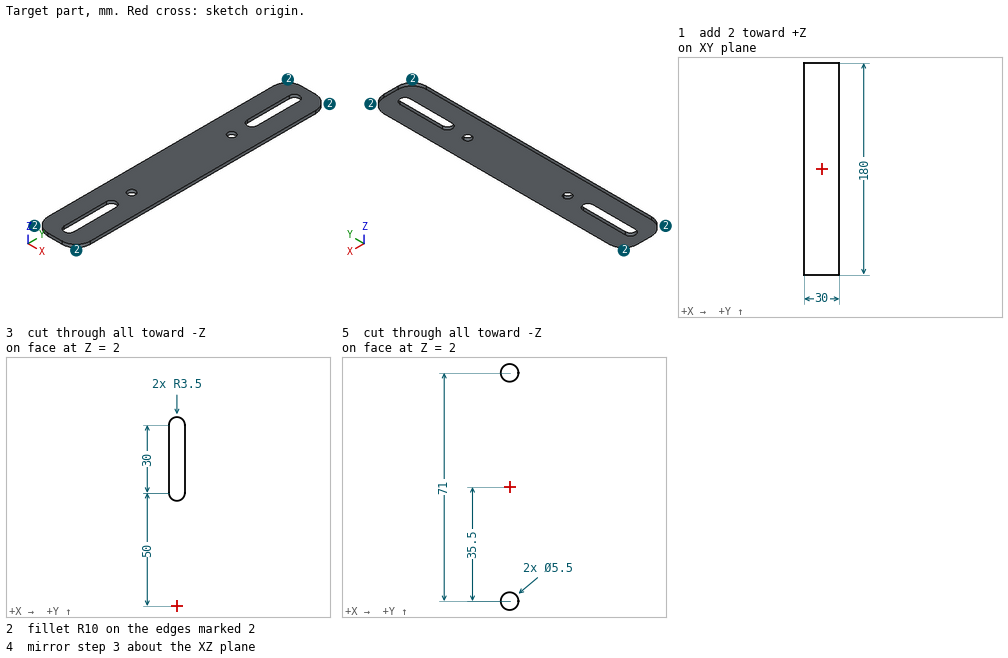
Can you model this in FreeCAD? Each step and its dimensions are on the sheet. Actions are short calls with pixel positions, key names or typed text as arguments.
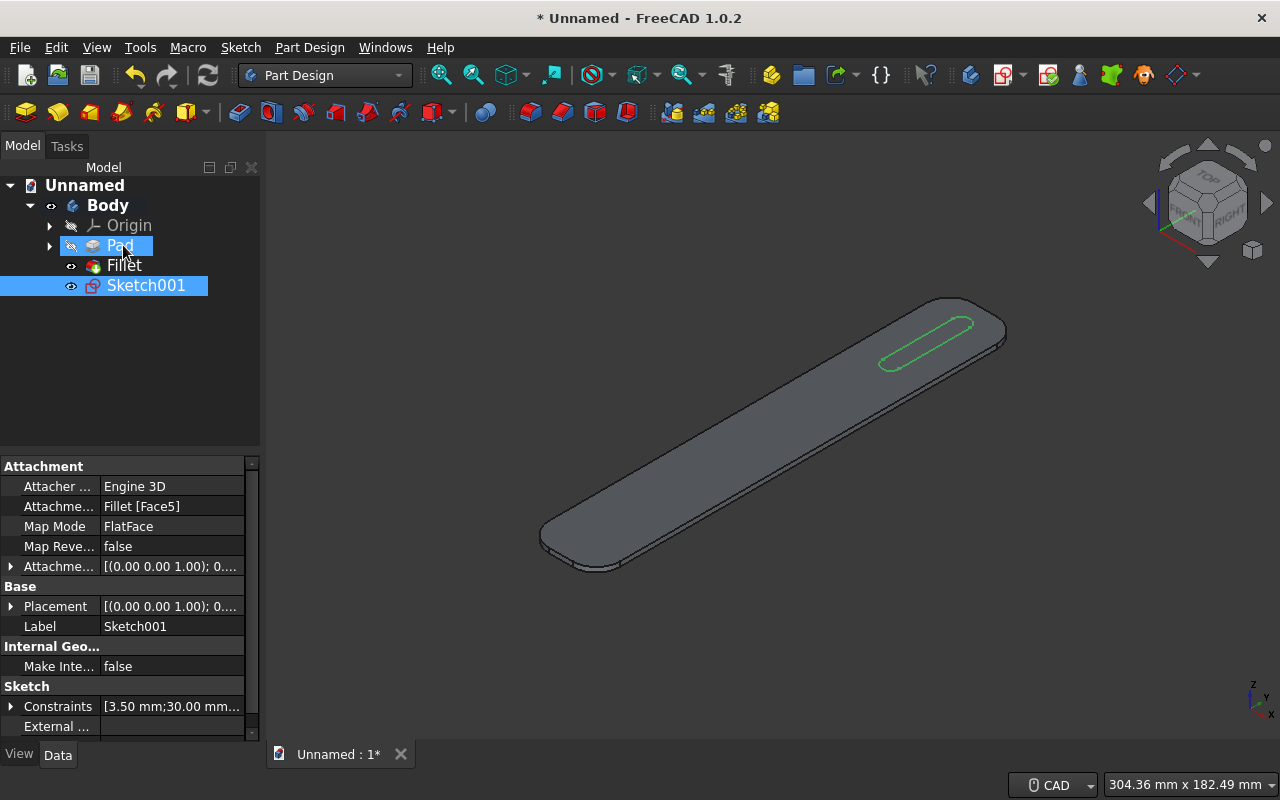
click(240, 112)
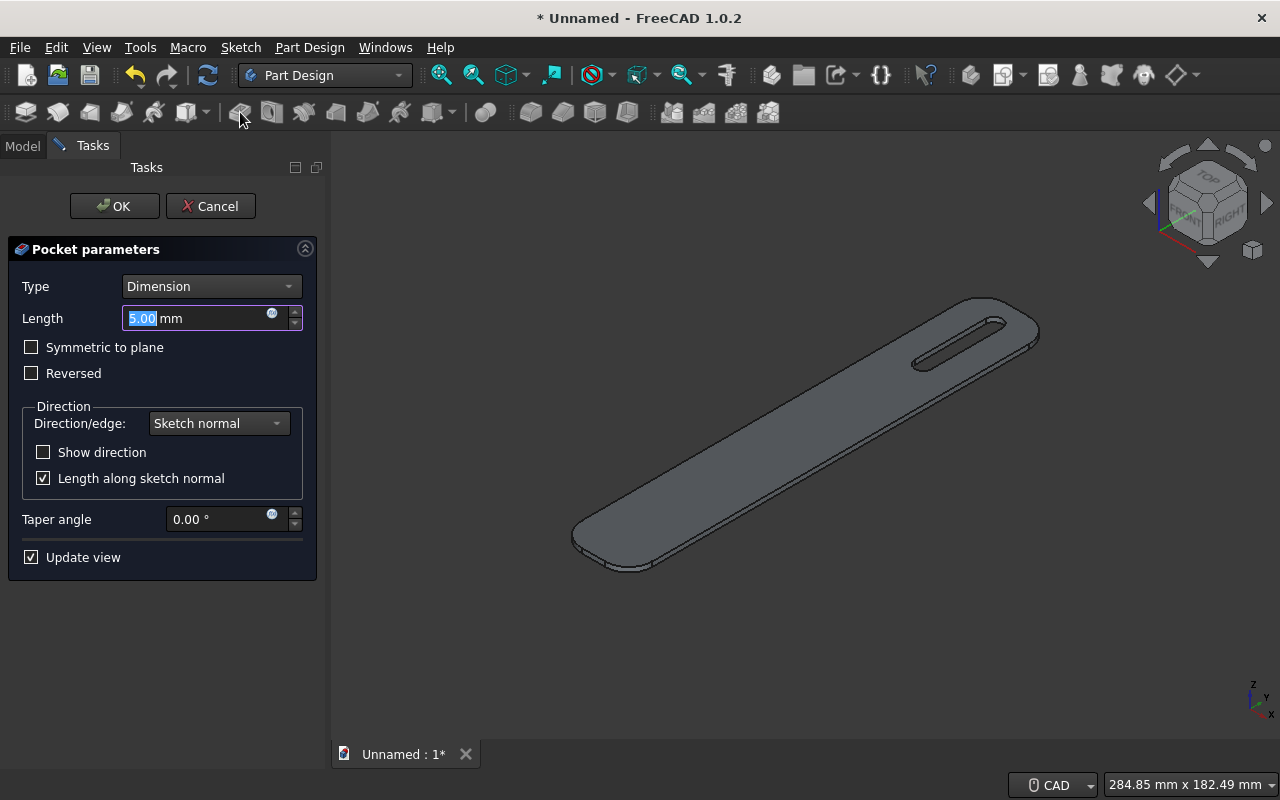
click(212, 286)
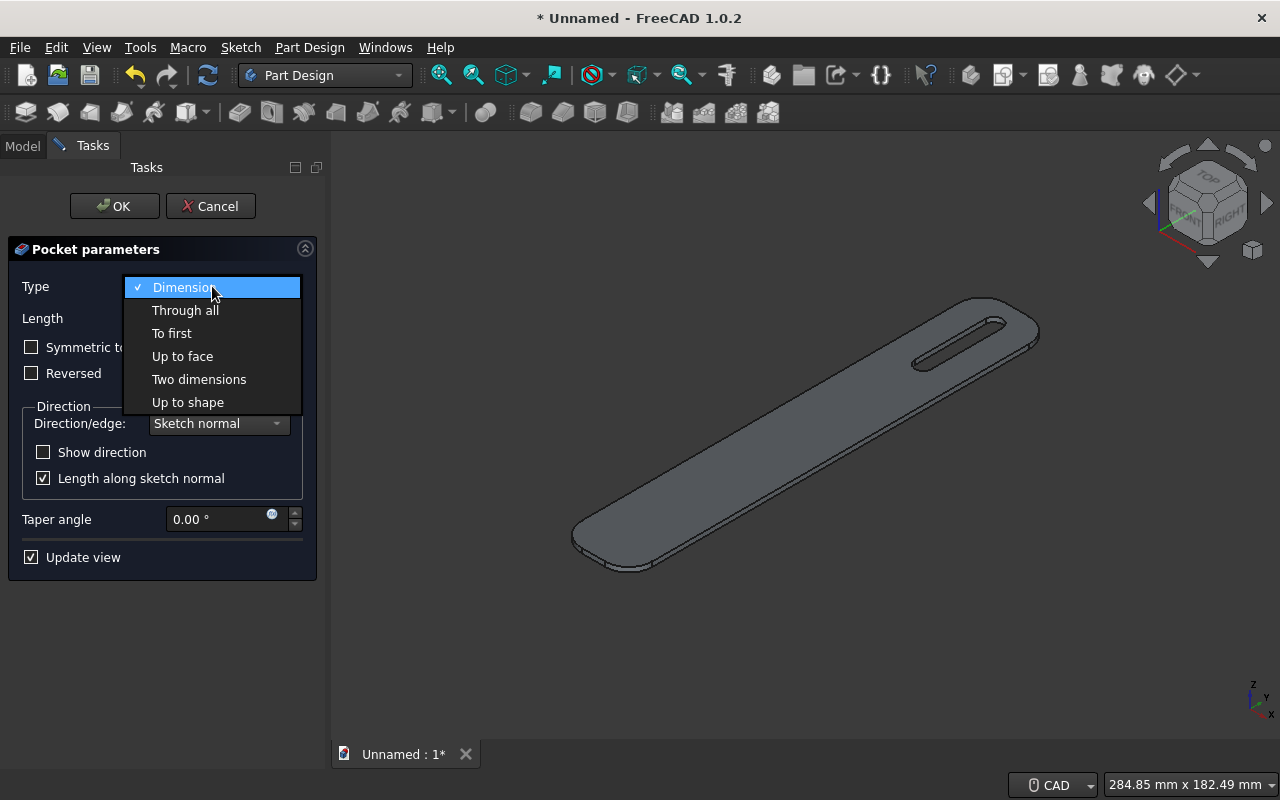
click(212, 310)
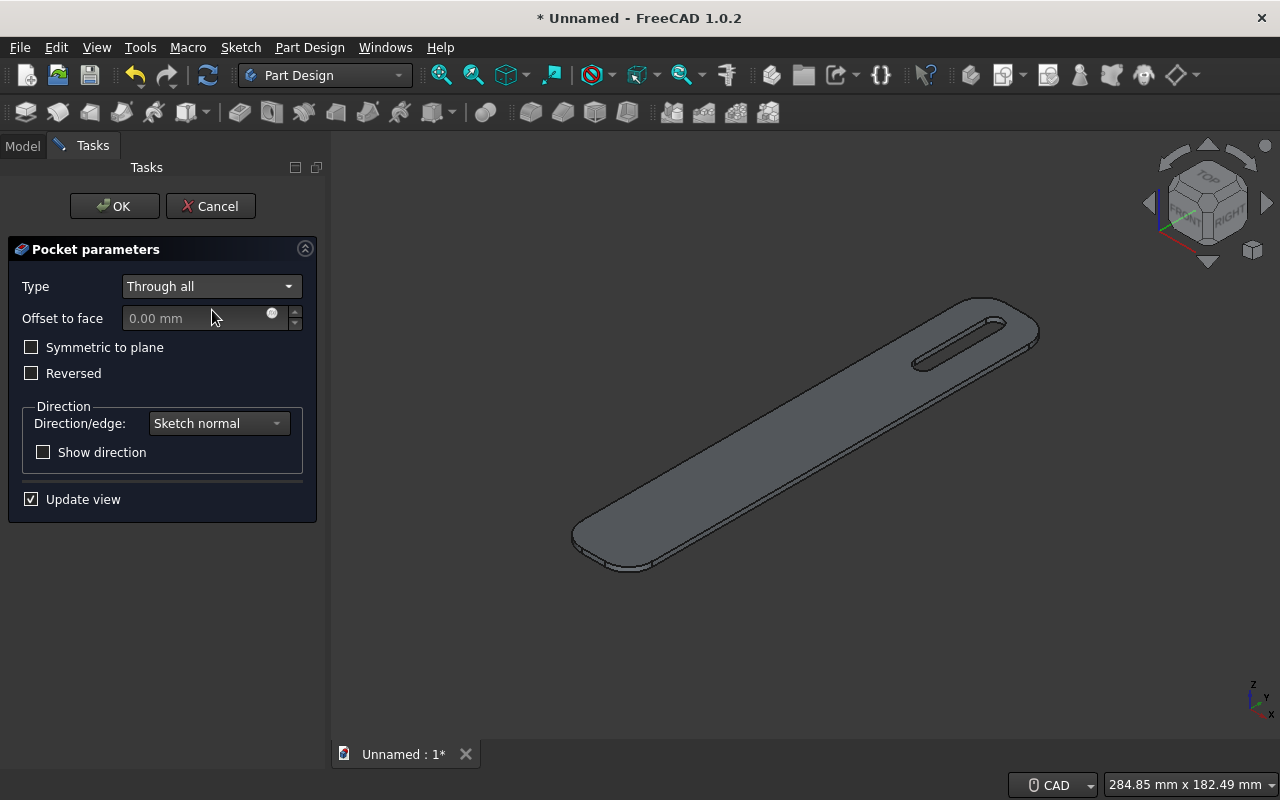
click(115, 206)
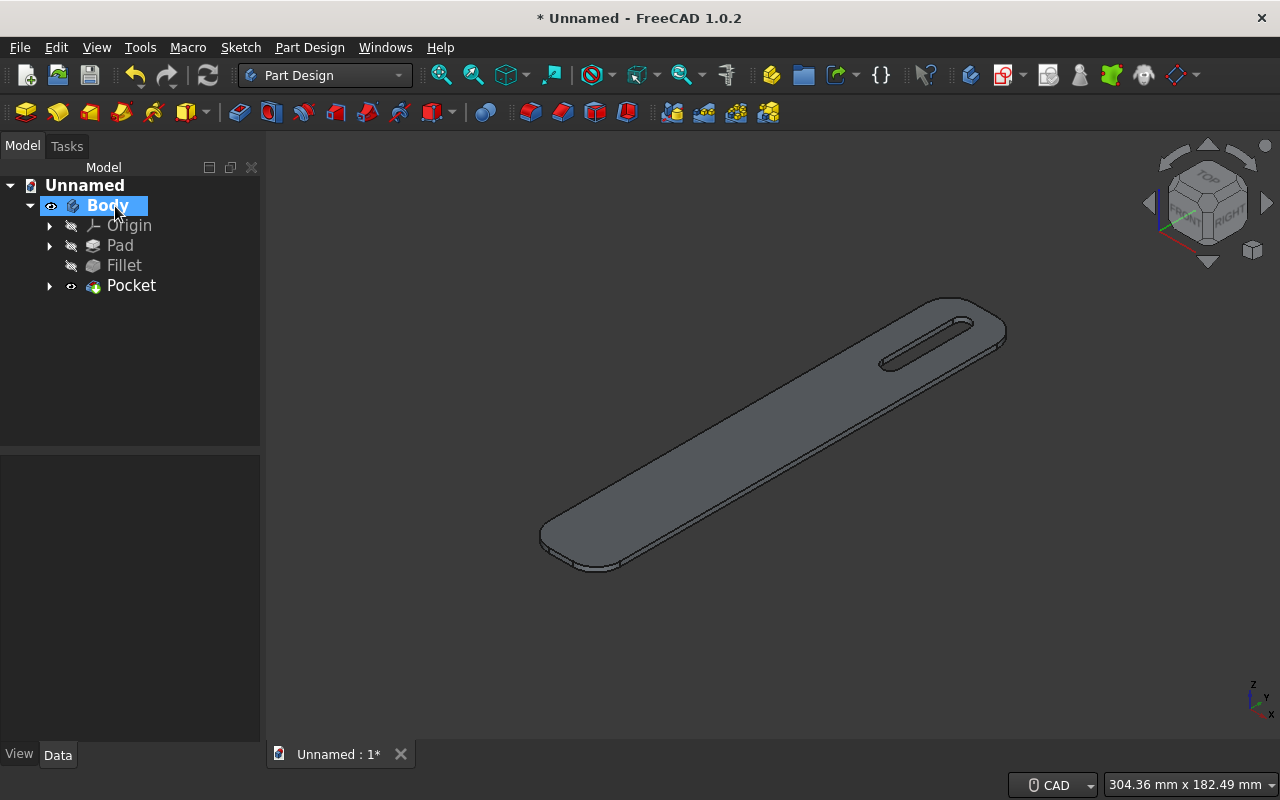
click(116, 286)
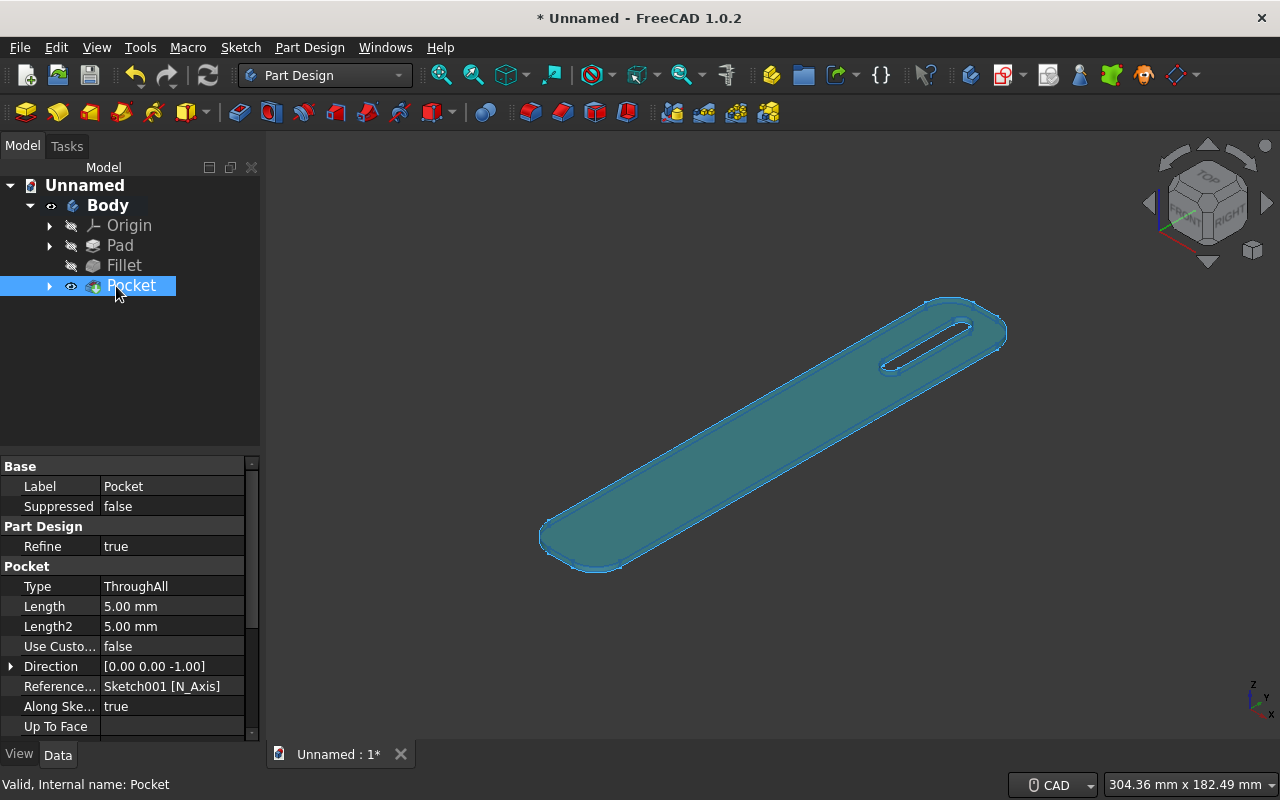
click(672, 112)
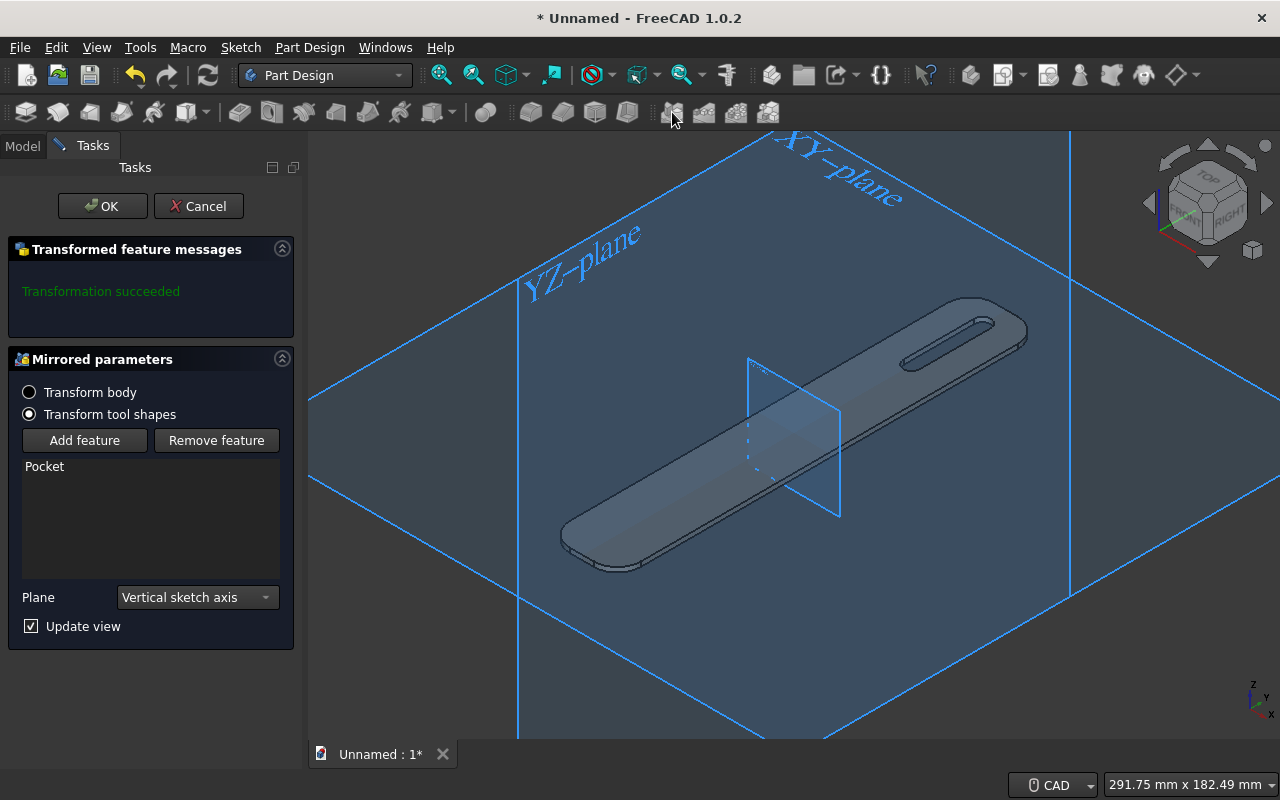
click(198, 598)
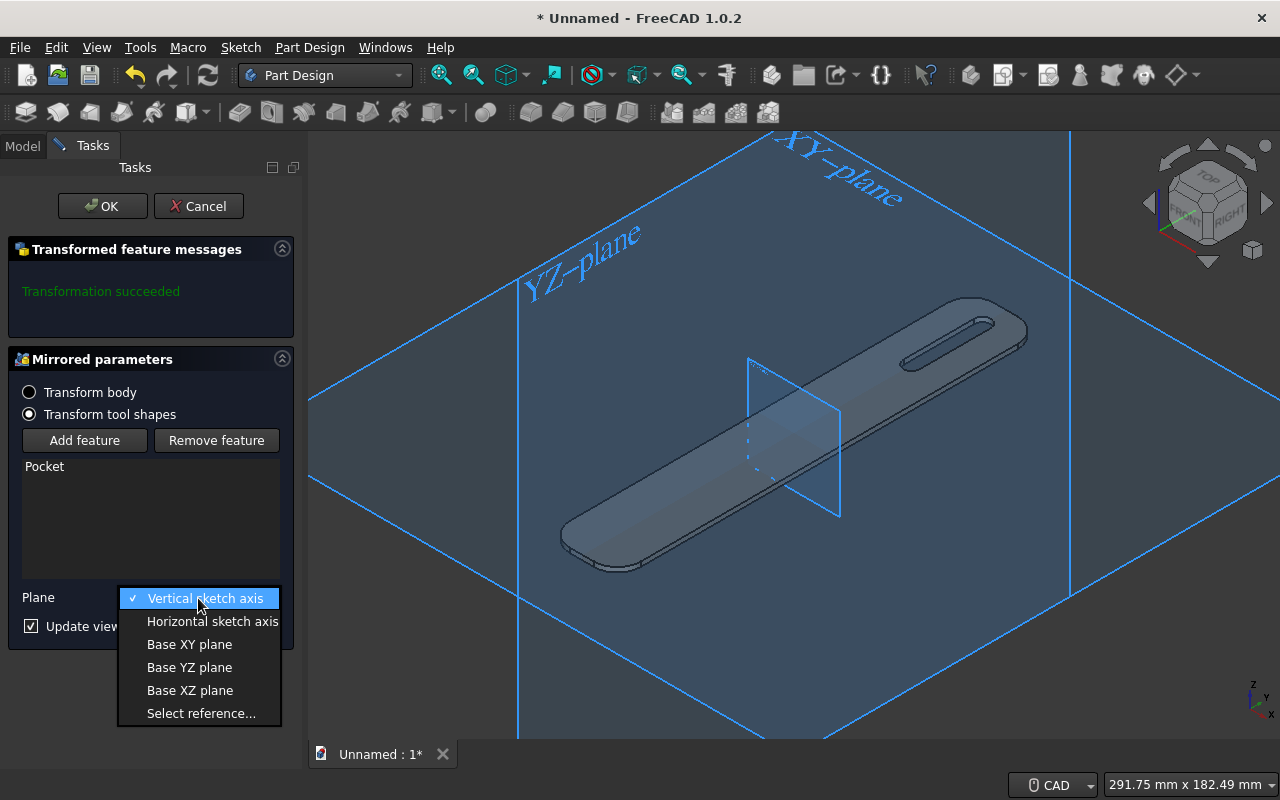
click(198, 690)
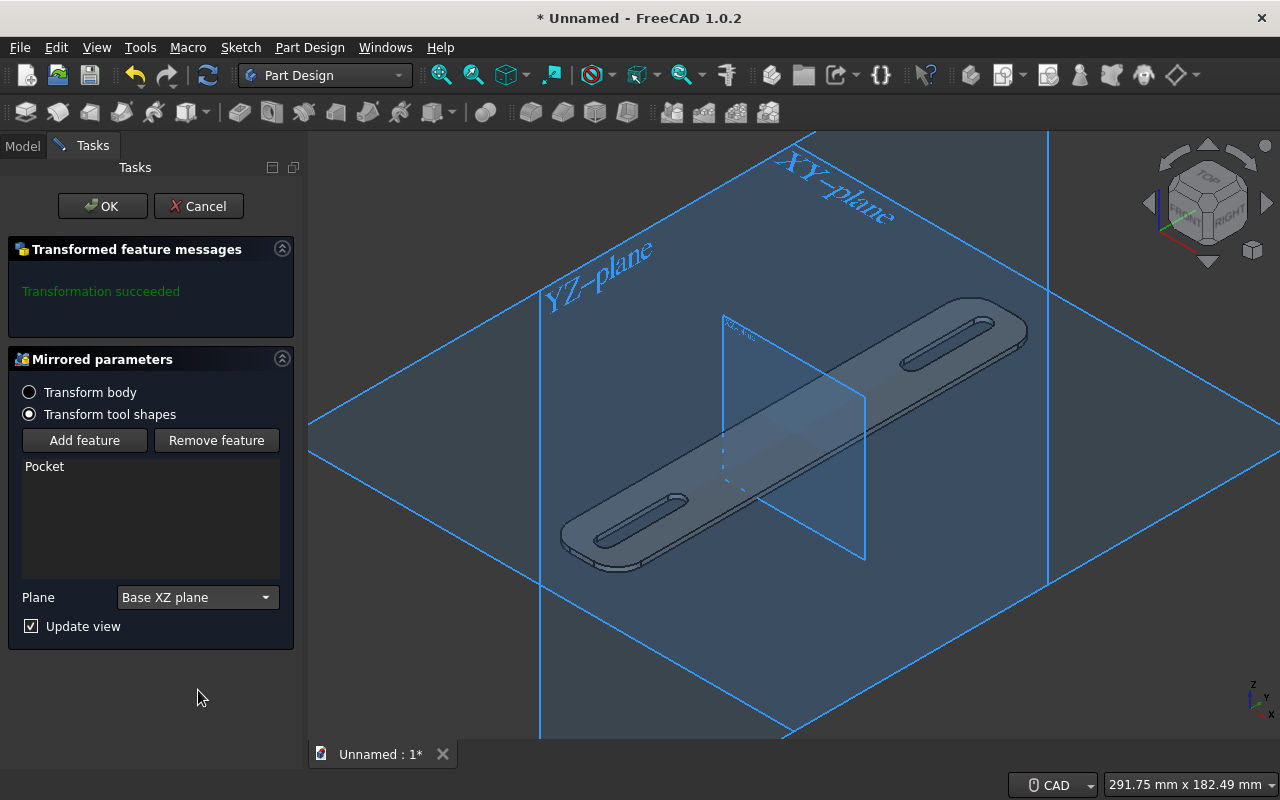
click(103, 206)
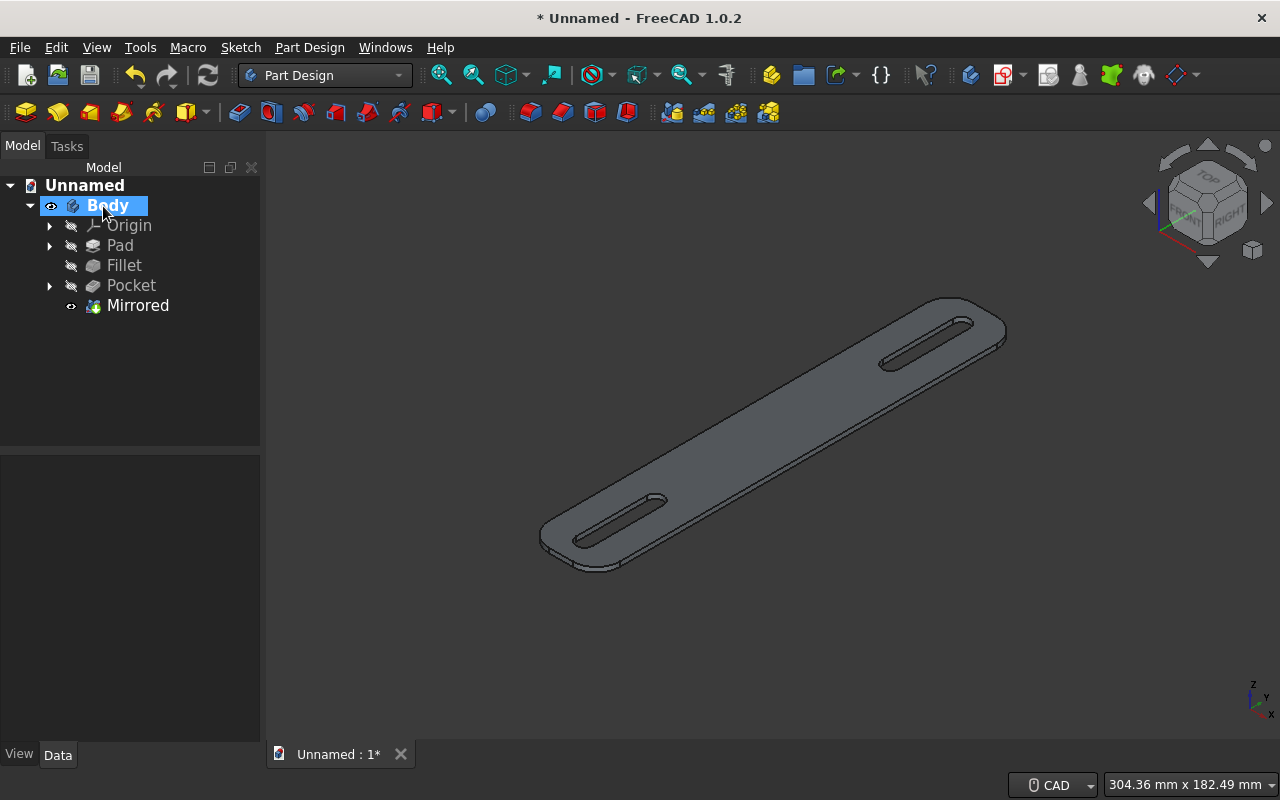
click(834, 396)